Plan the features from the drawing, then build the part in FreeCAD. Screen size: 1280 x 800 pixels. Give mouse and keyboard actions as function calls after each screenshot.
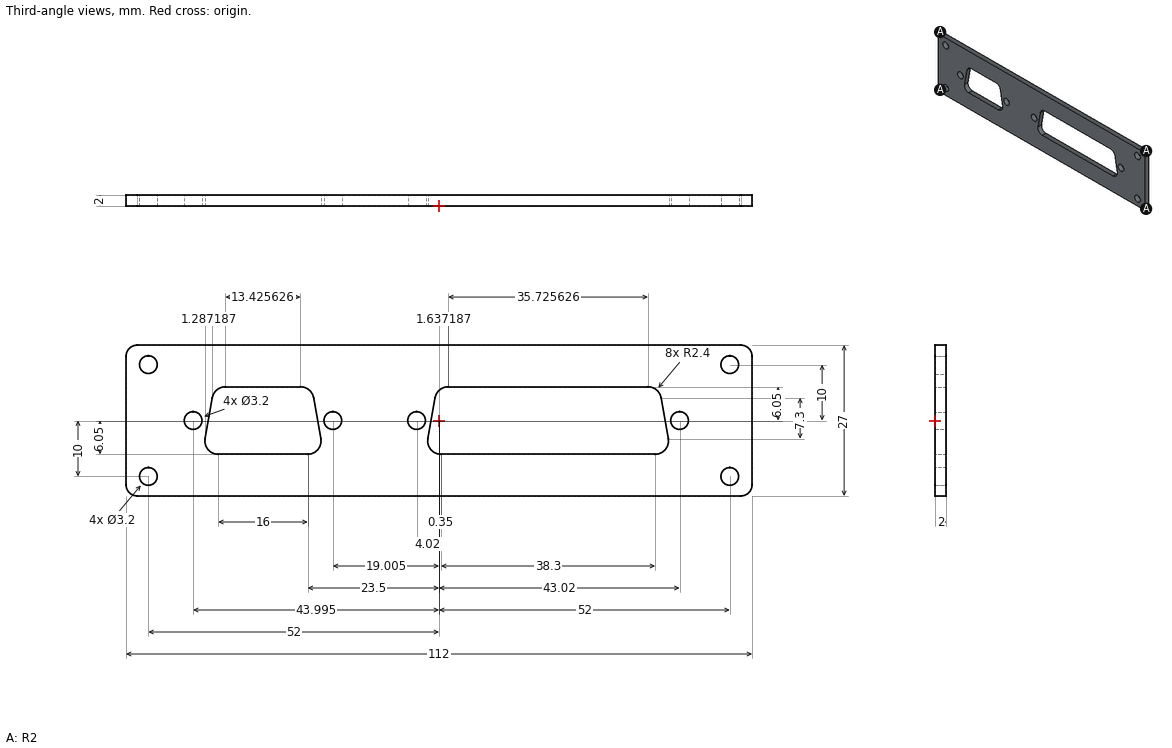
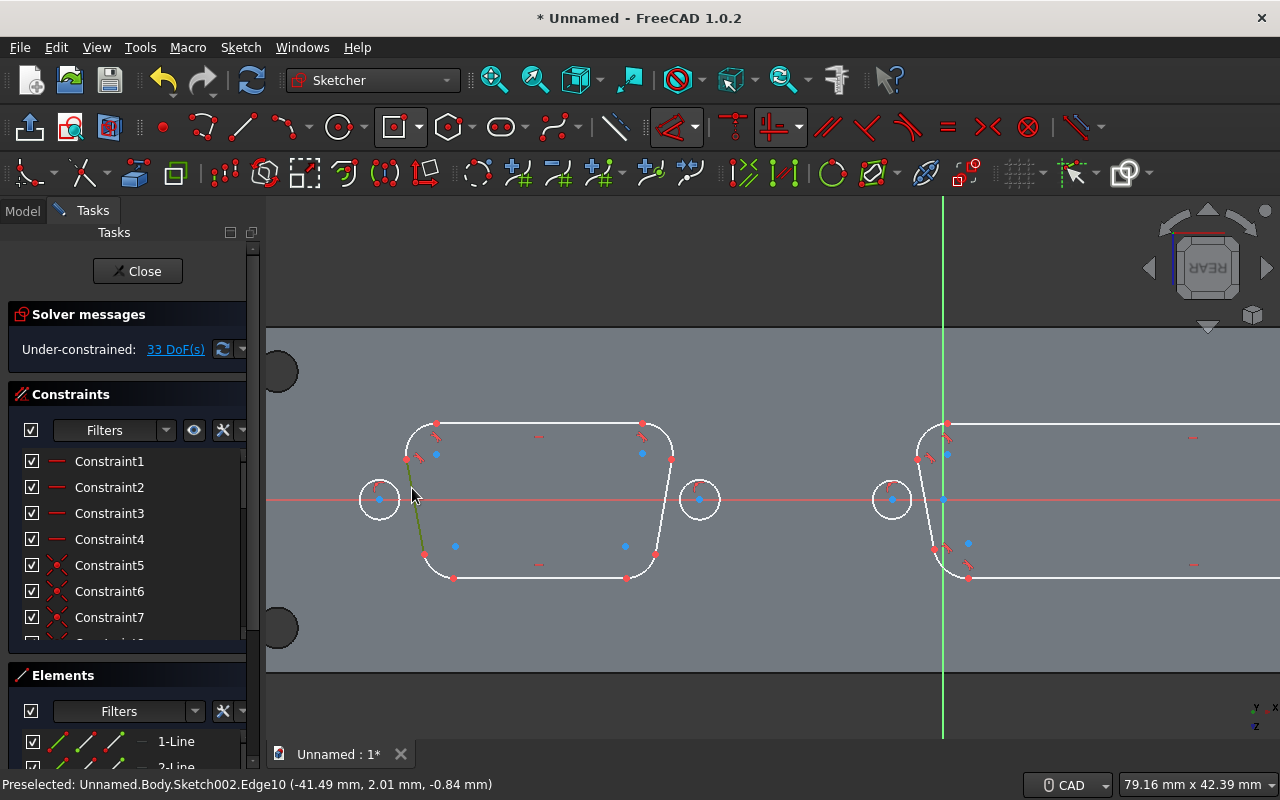
click(429, 565)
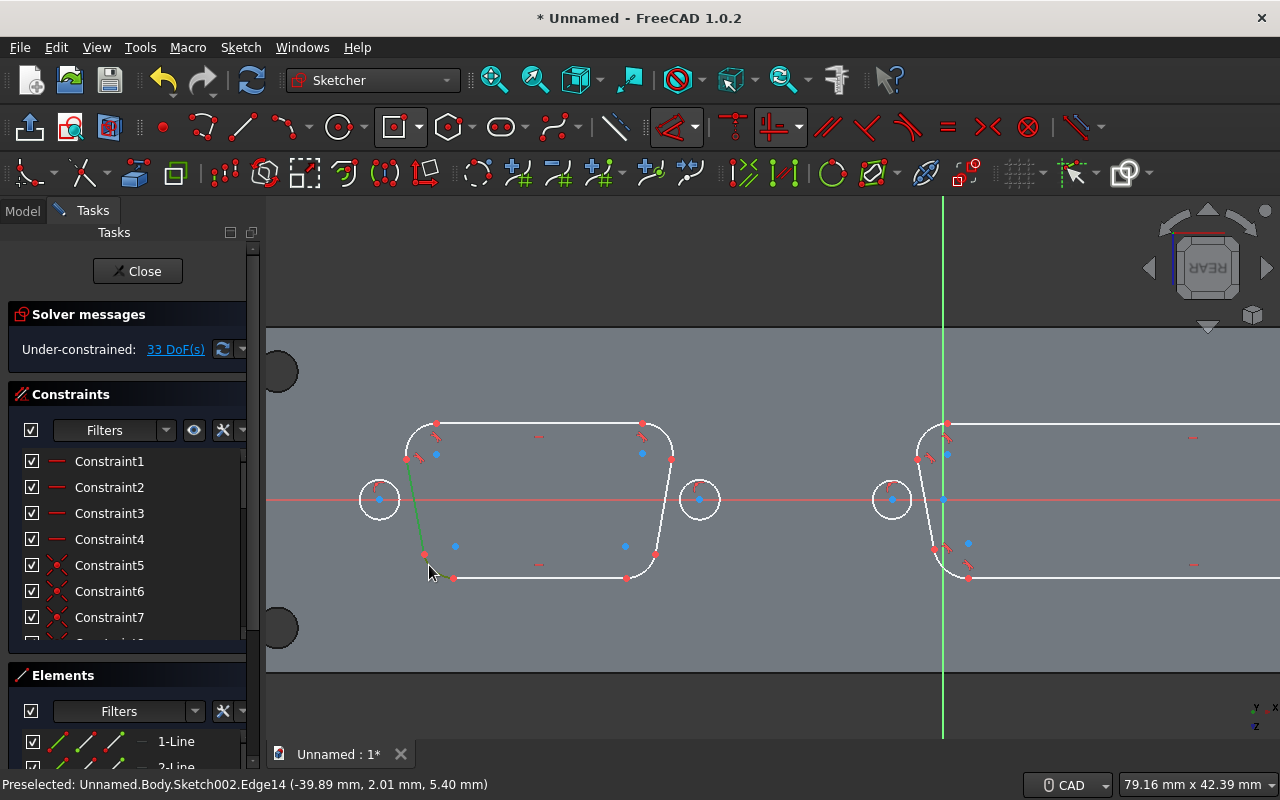
click(908, 128)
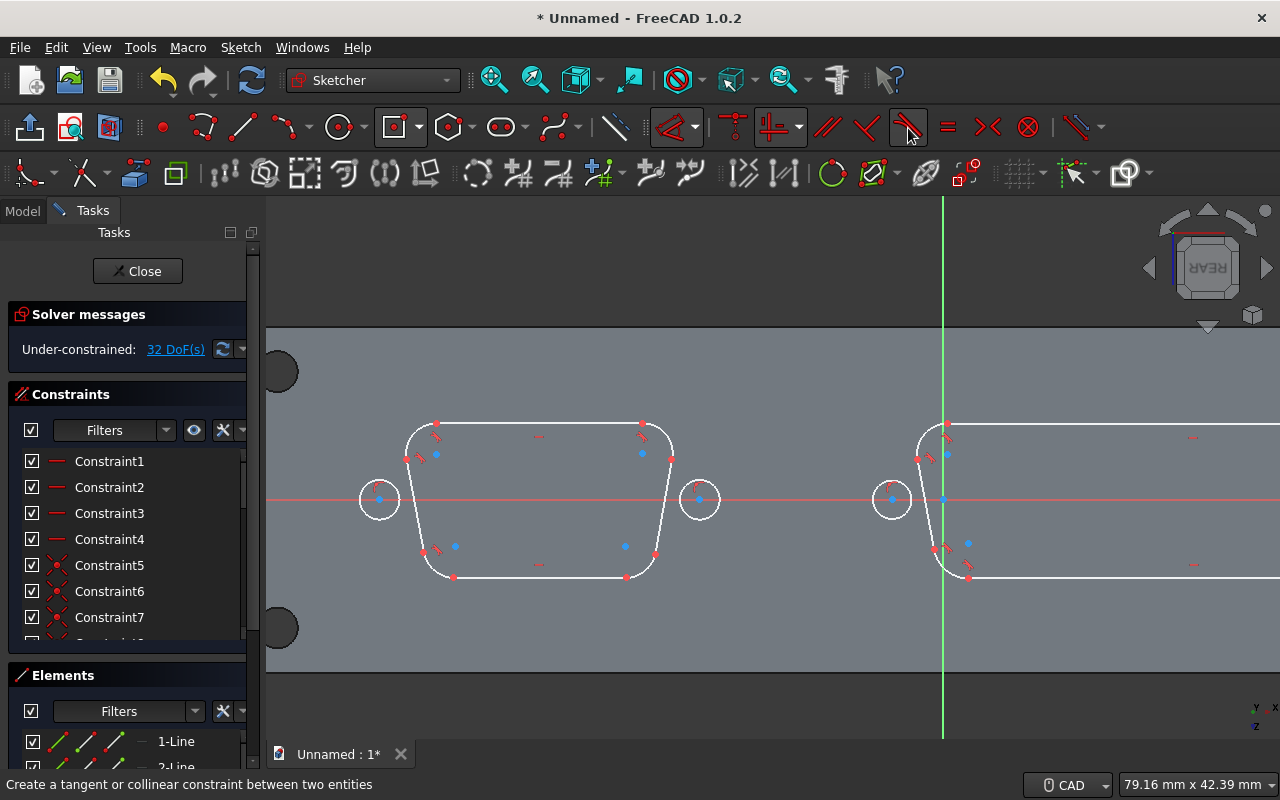
click(505, 578)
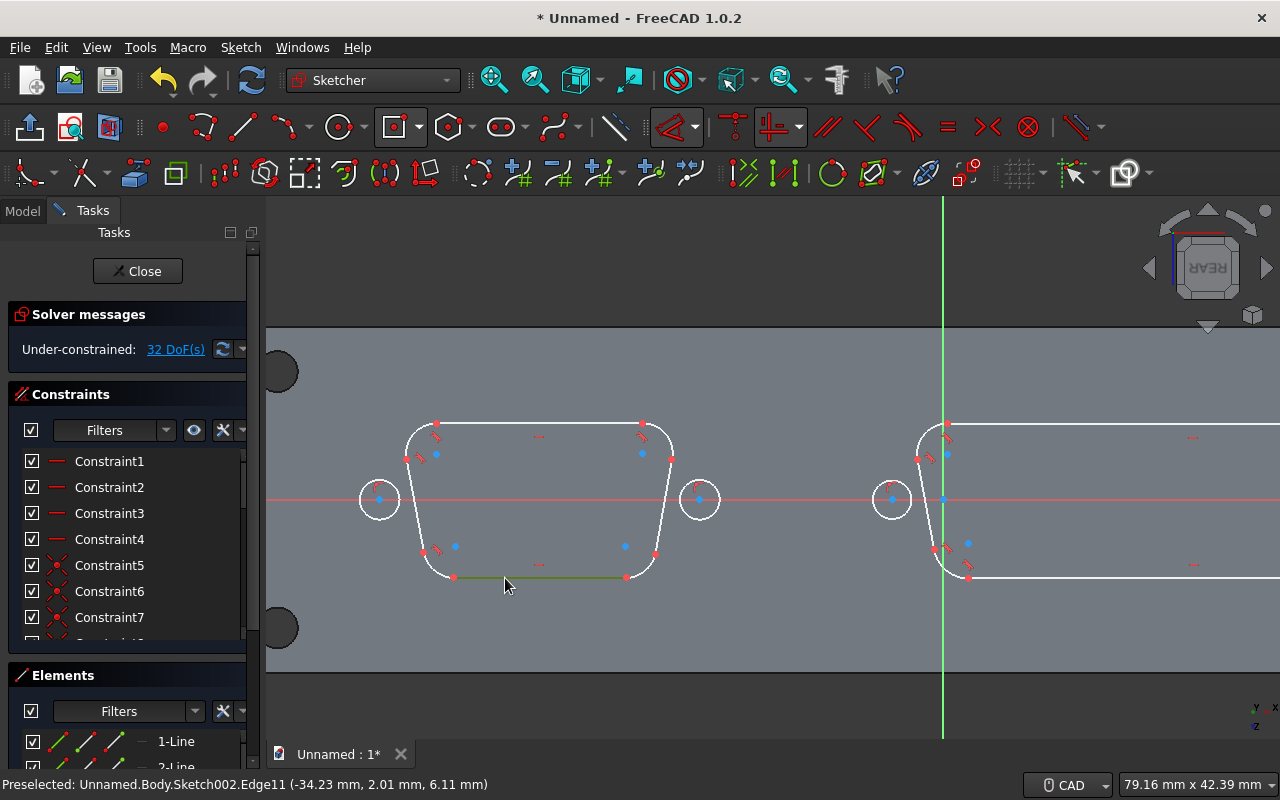
click(429, 564)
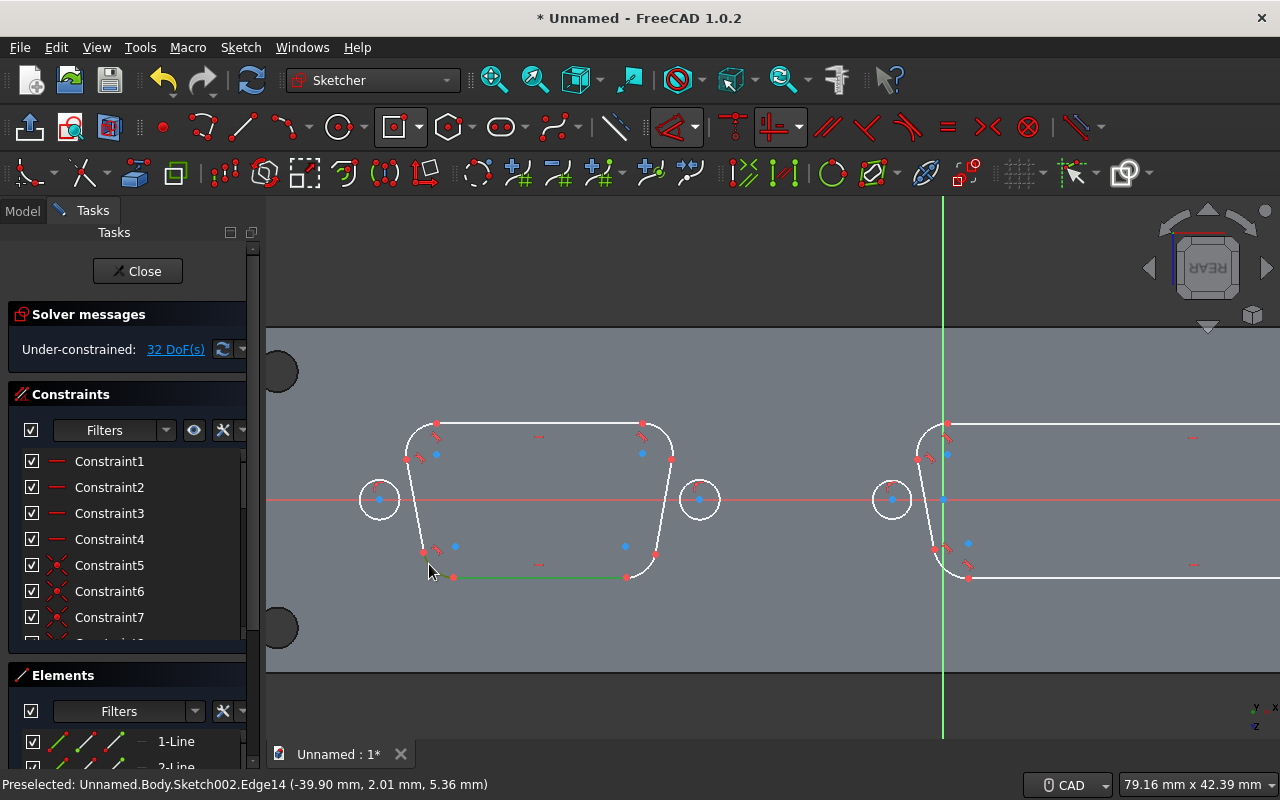
key(t)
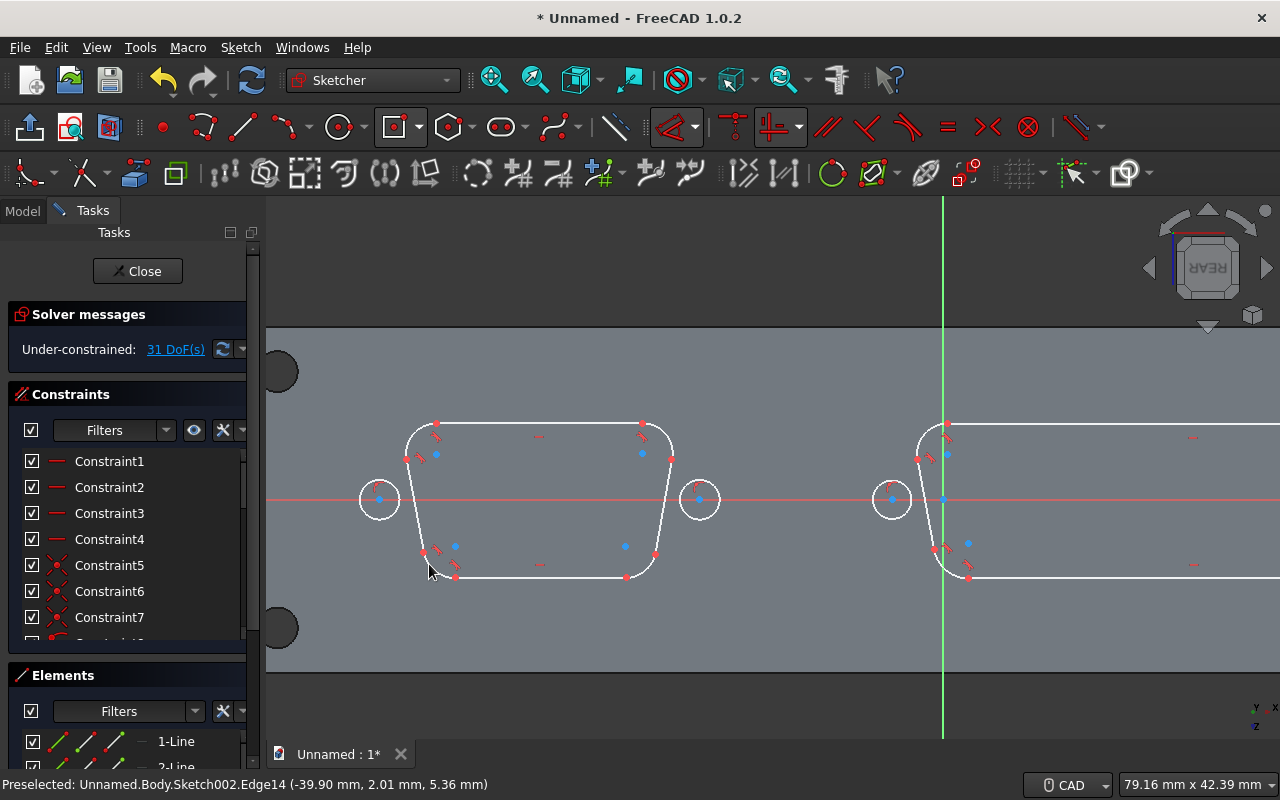
click(506, 578)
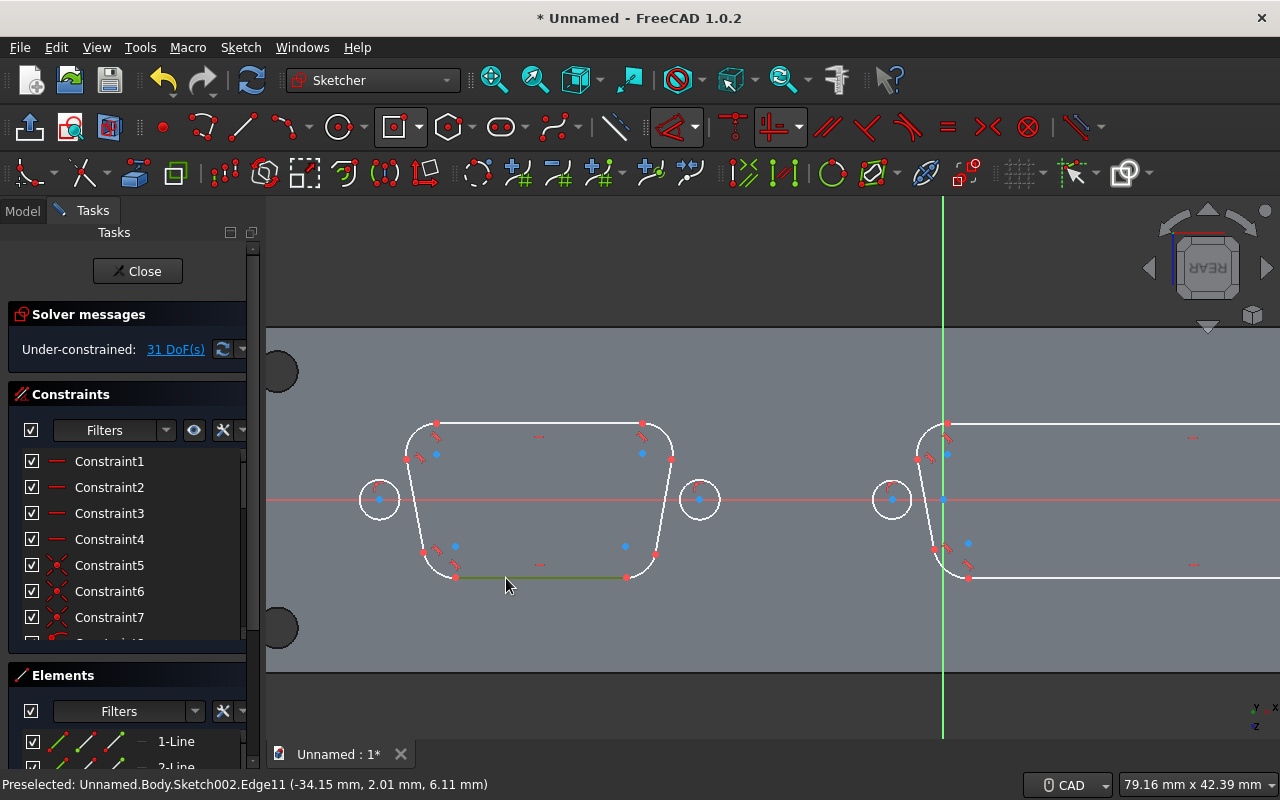
click(638, 575)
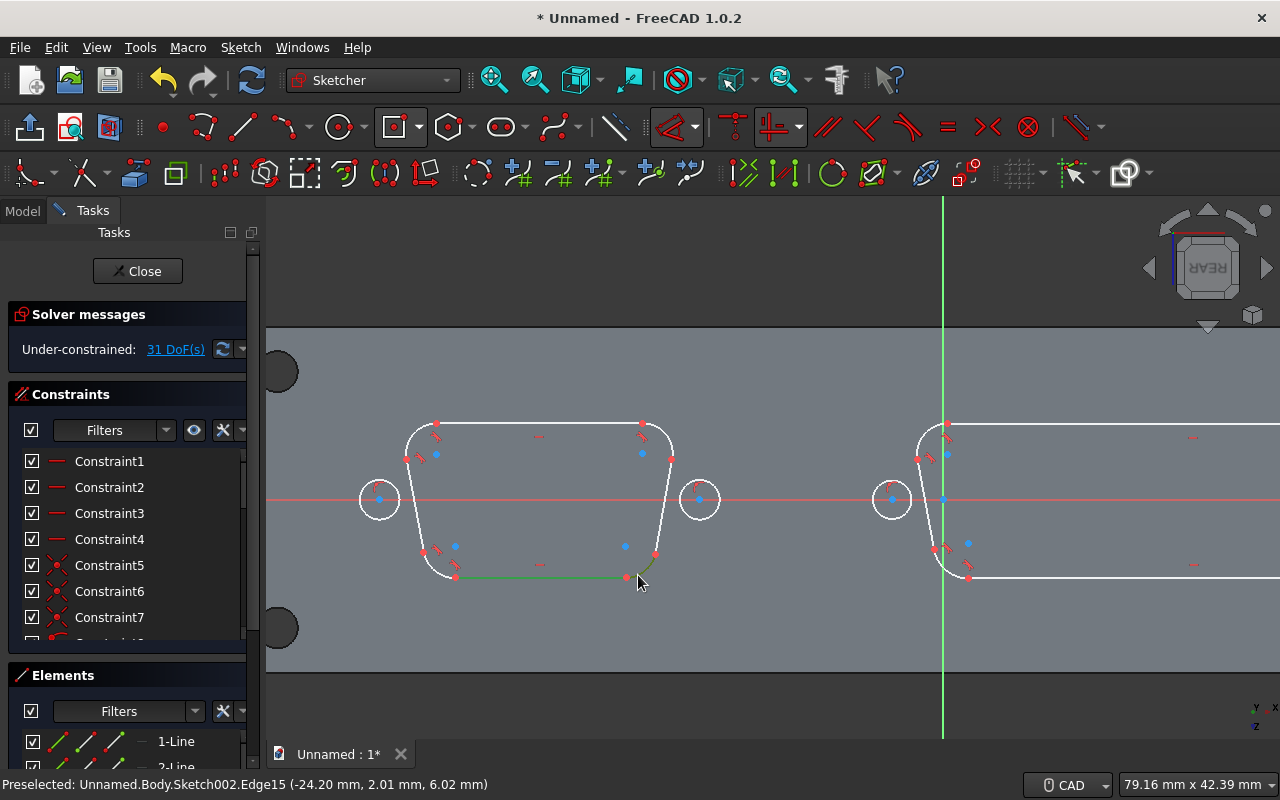
click(908, 128)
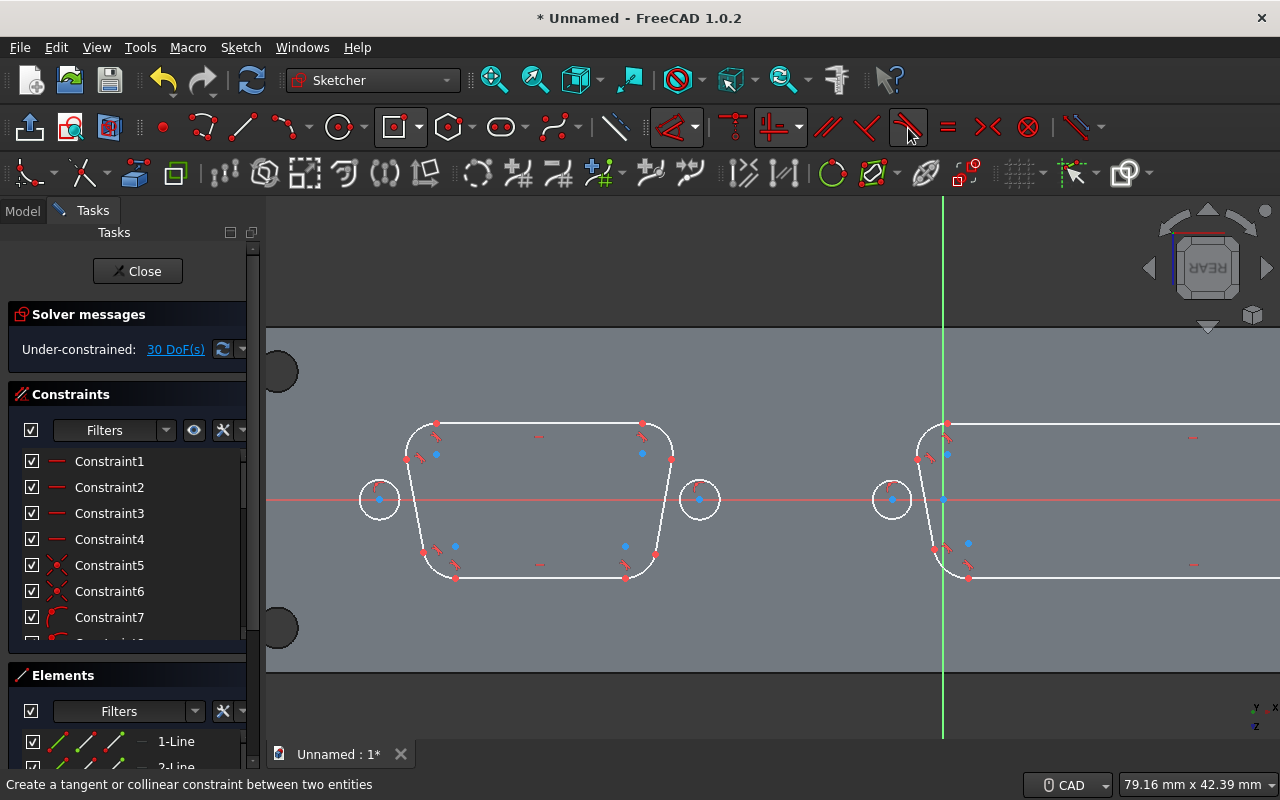
click(660, 526)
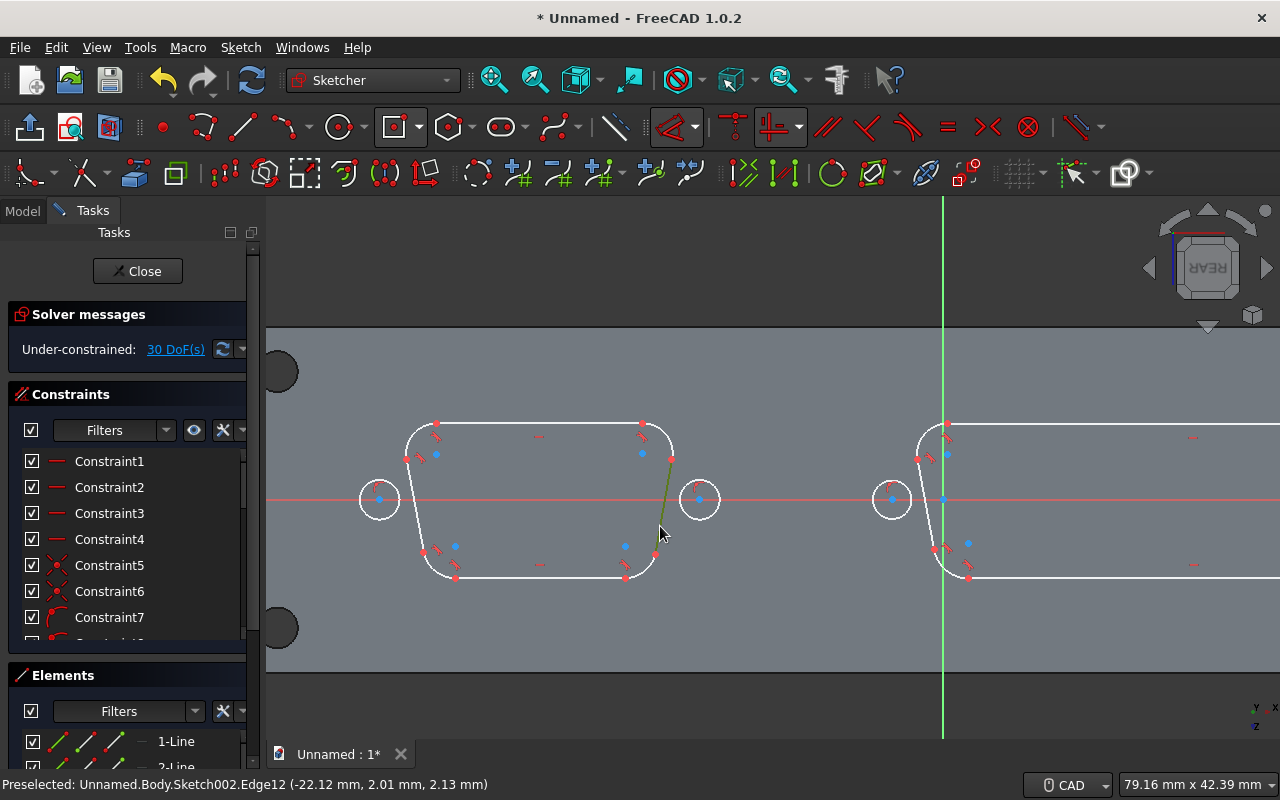
click(637, 576)